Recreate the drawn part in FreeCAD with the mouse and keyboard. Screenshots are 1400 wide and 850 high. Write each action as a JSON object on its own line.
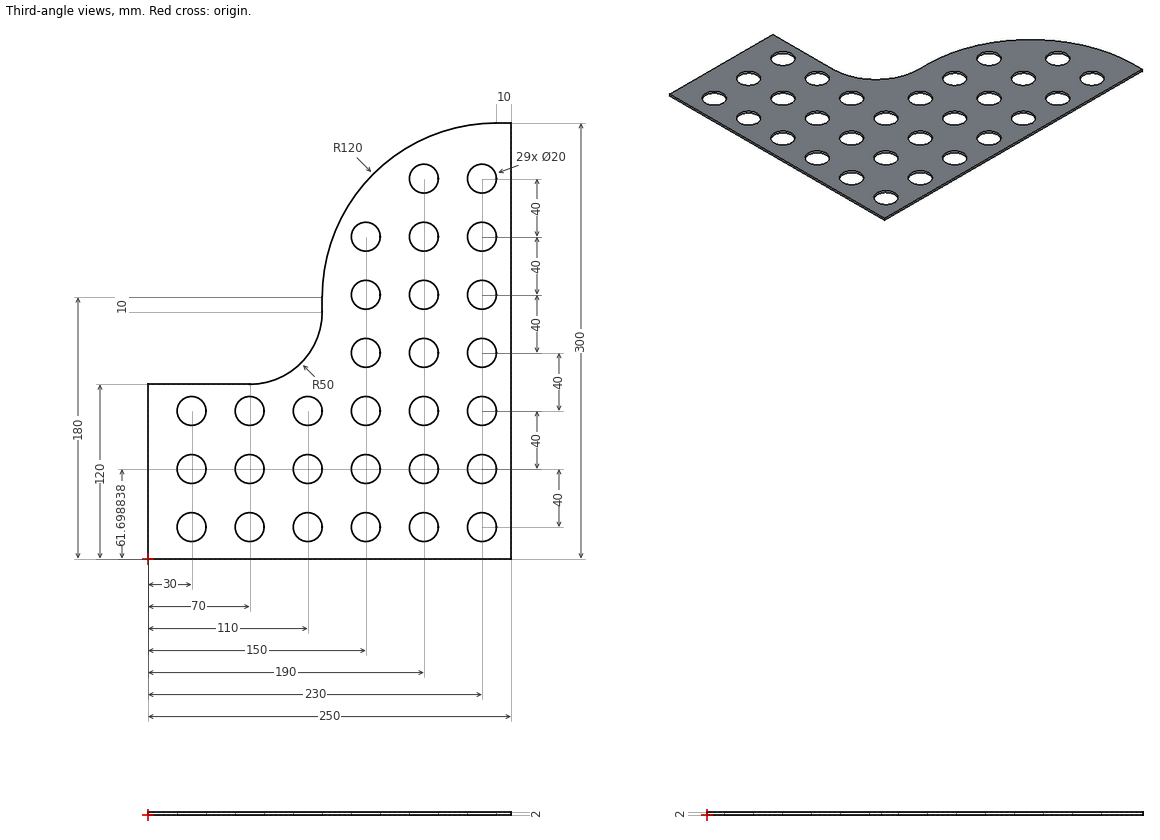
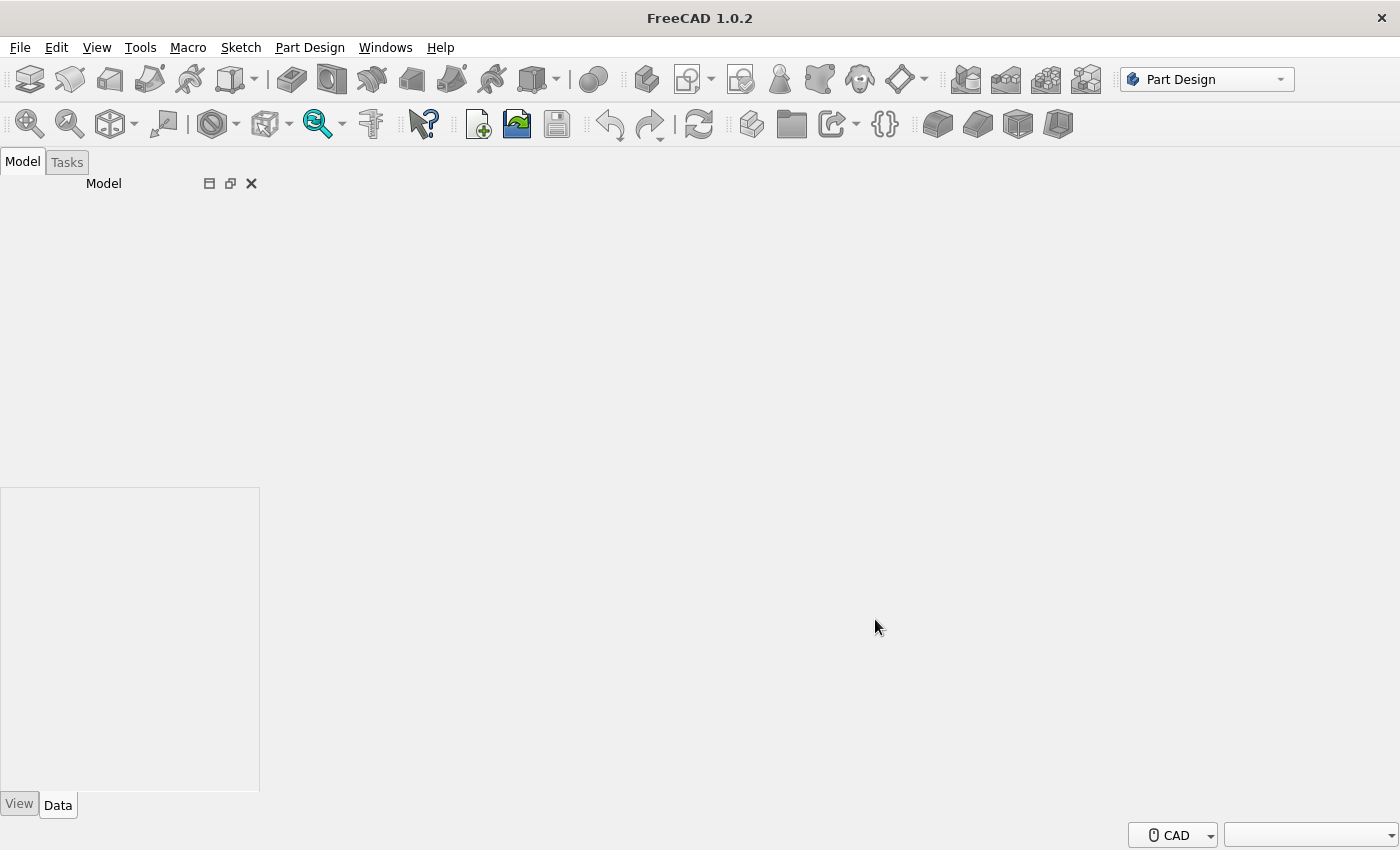
{"action": "left_click", "coordinate": [478, 124]}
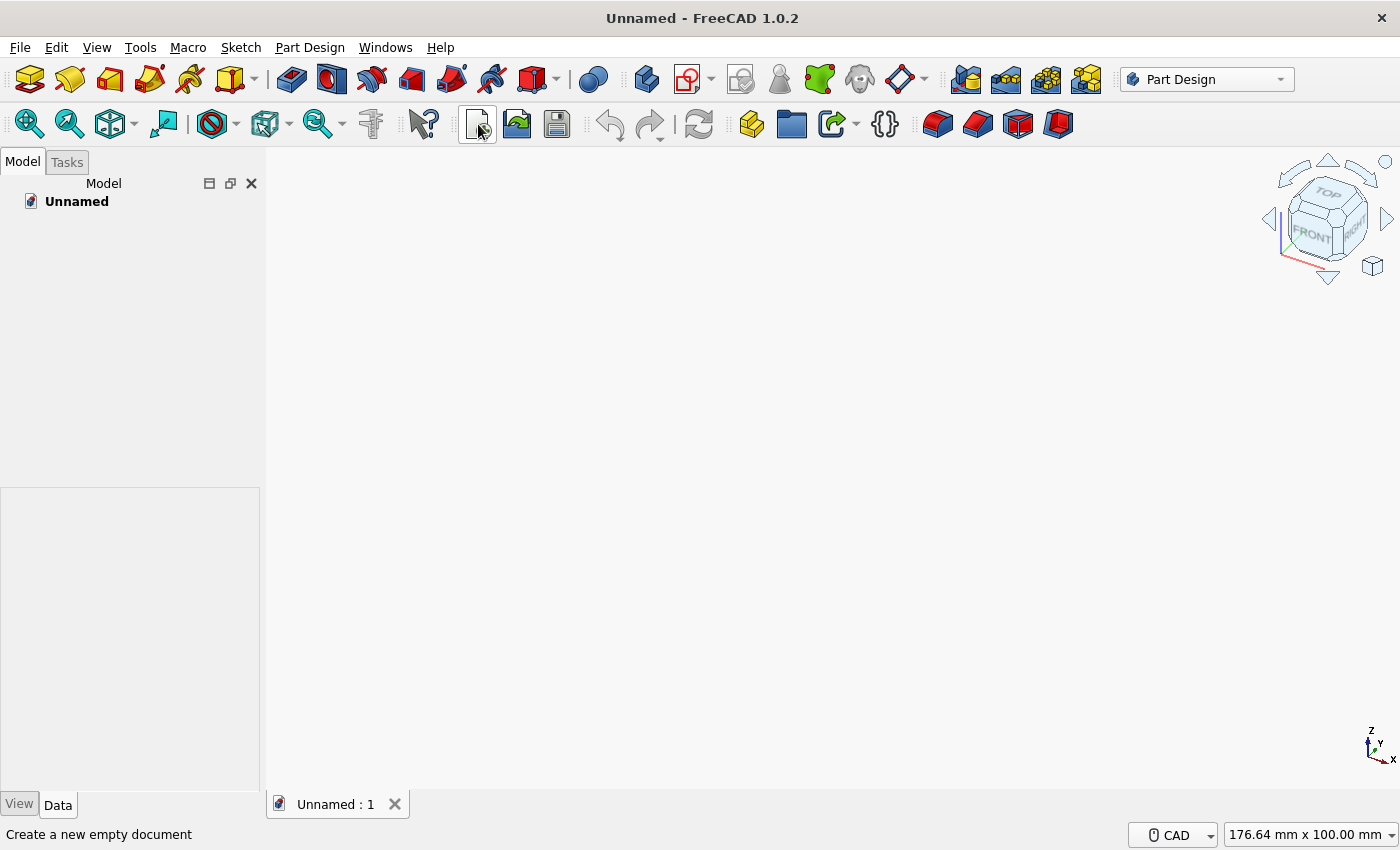
{"action": "left_click", "coordinate": [688, 80]}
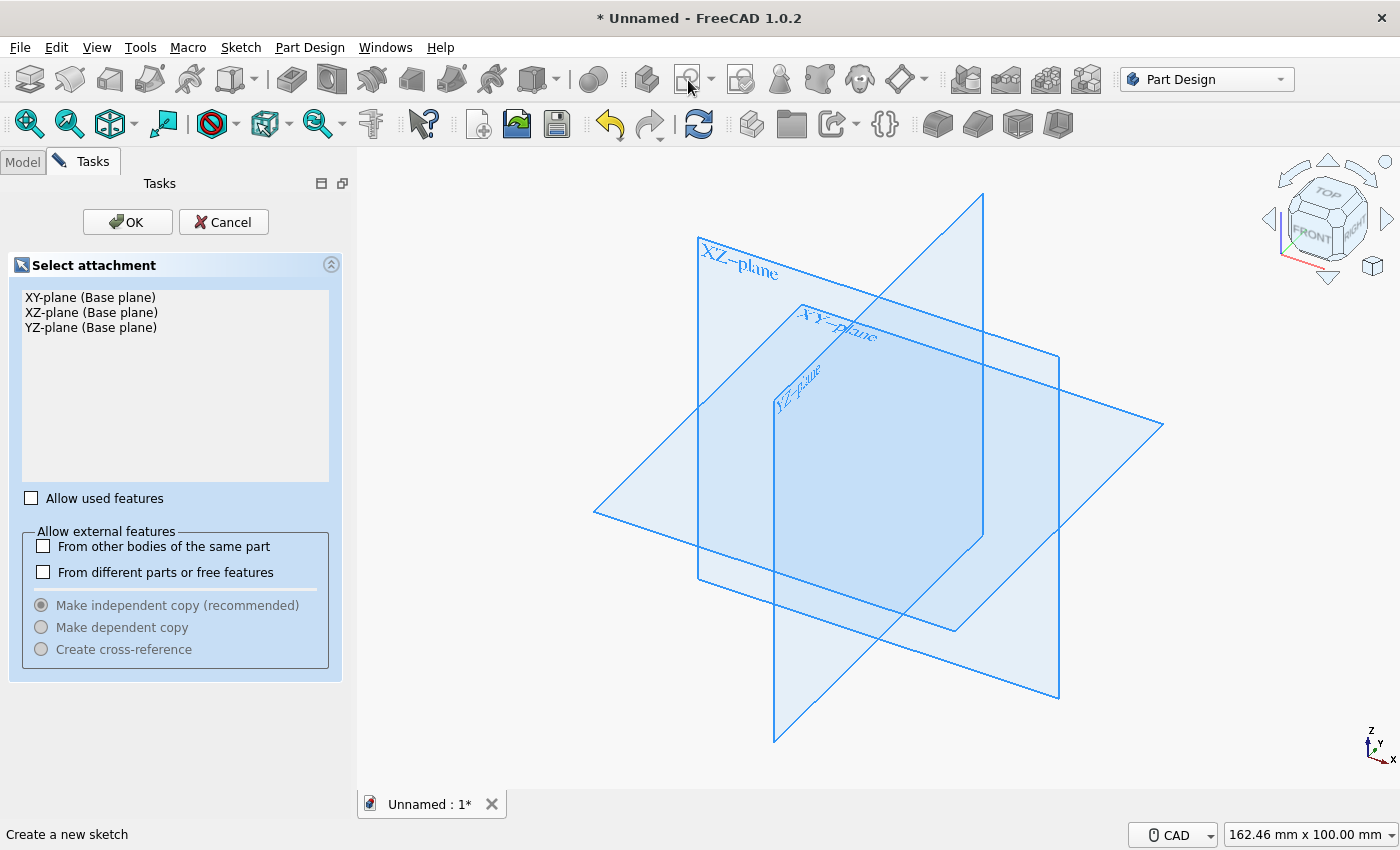
{"action": "left_click", "coordinate": [82, 298]}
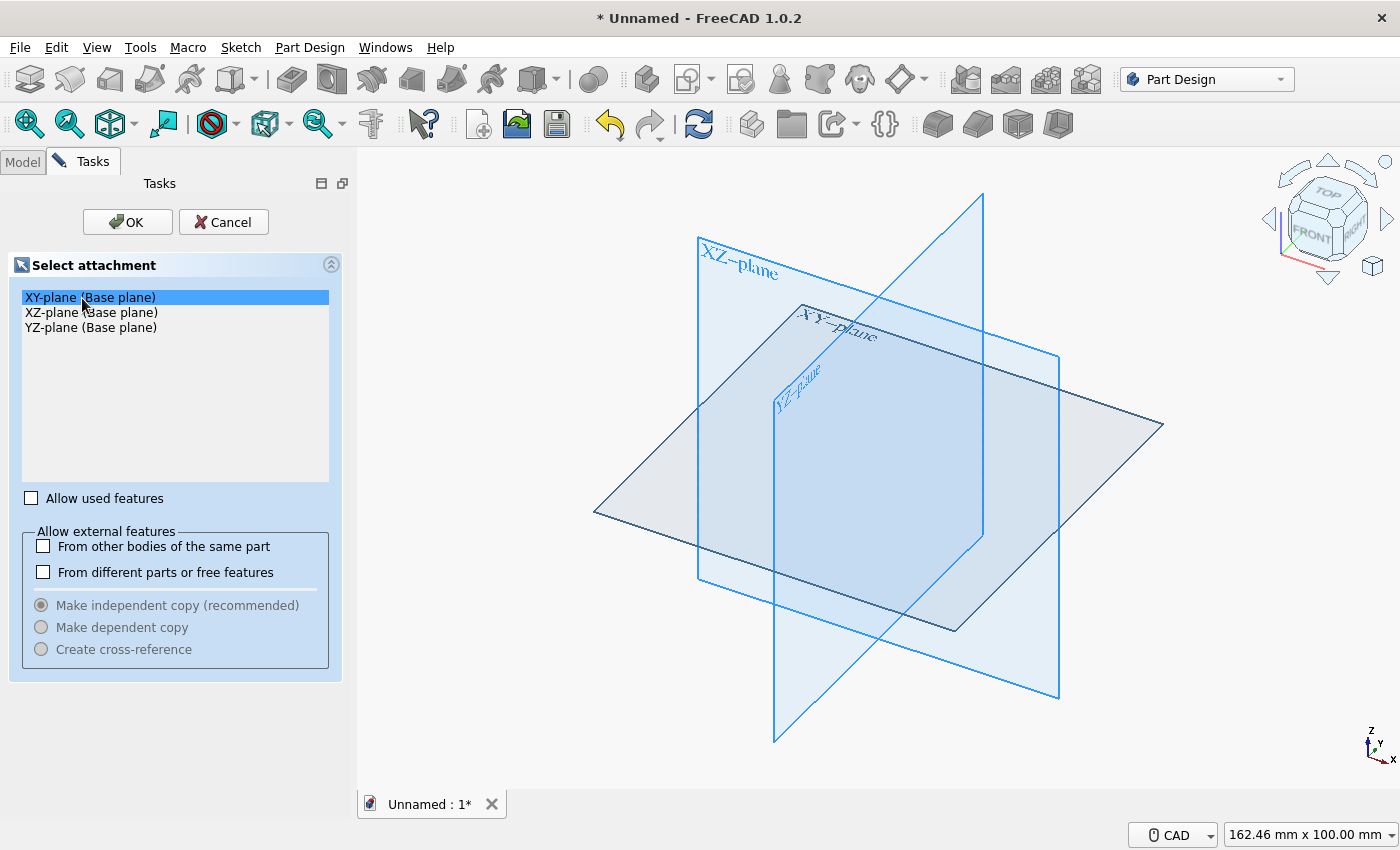
{"action": "left_click", "coordinate": [128, 222]}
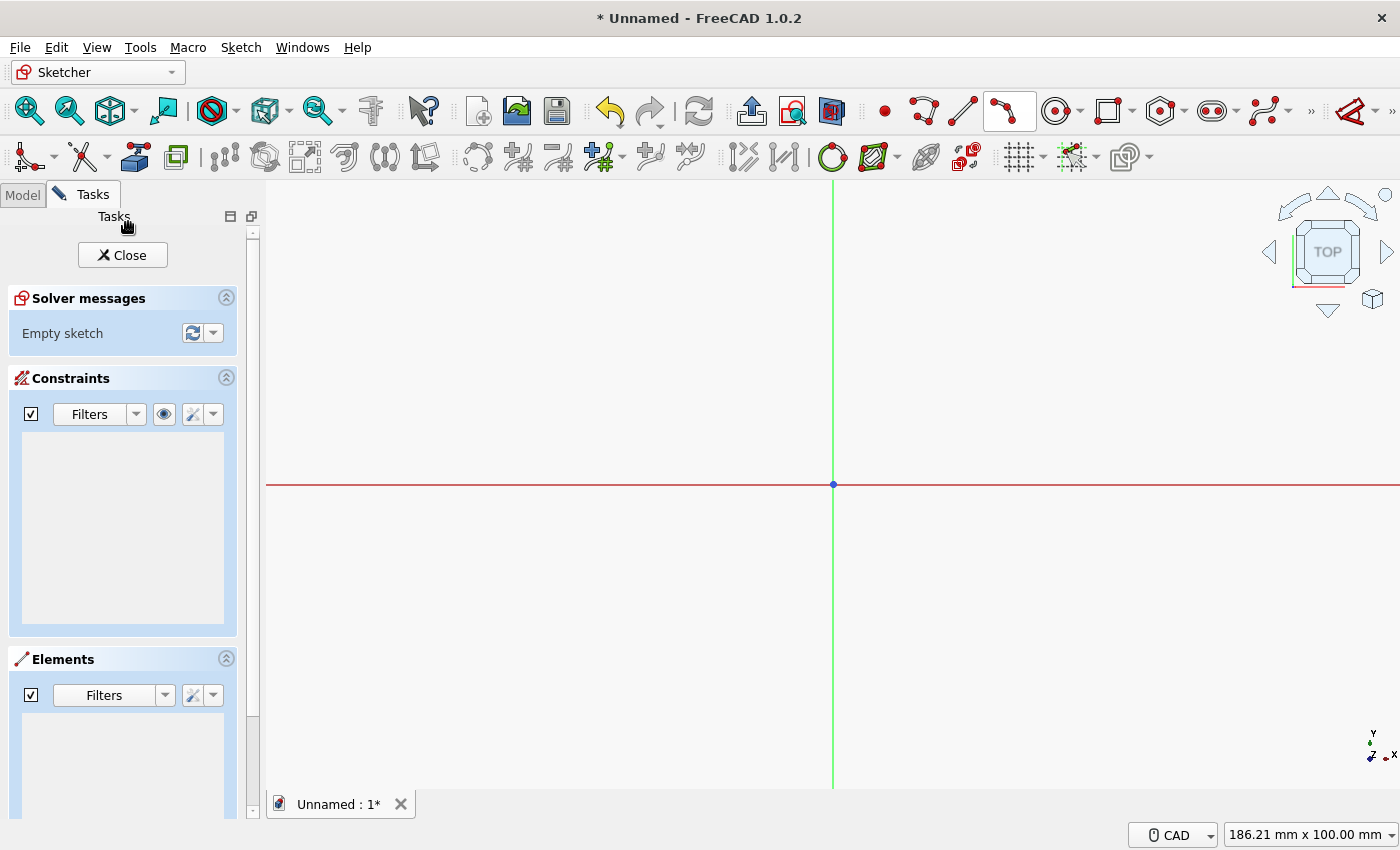
{"action": "scroll", "coordinate": [555, 716], "scroll_direction": "down", "scroll_amount": 8}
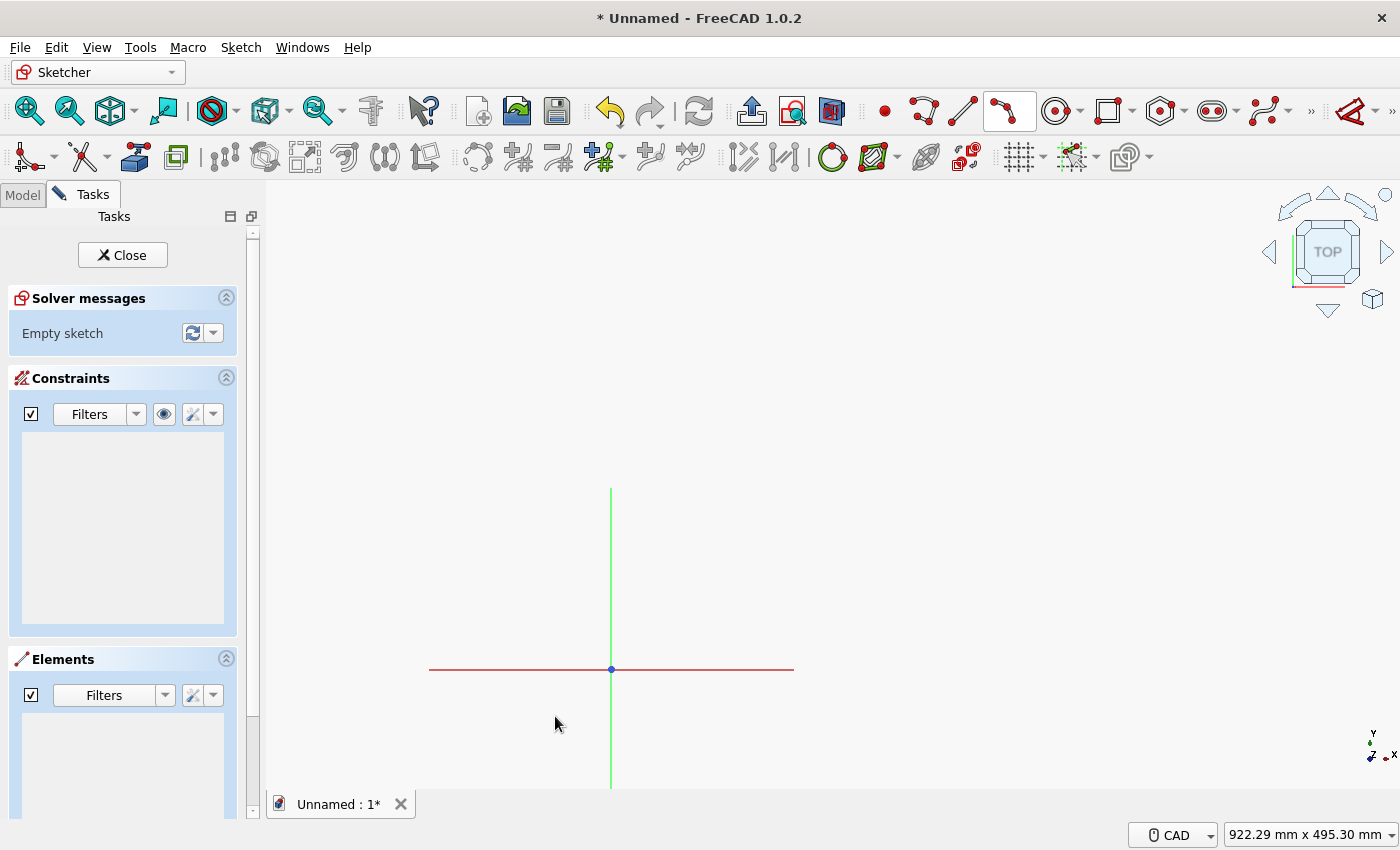
{"action": "left_click", "coordinate": [964, 112]}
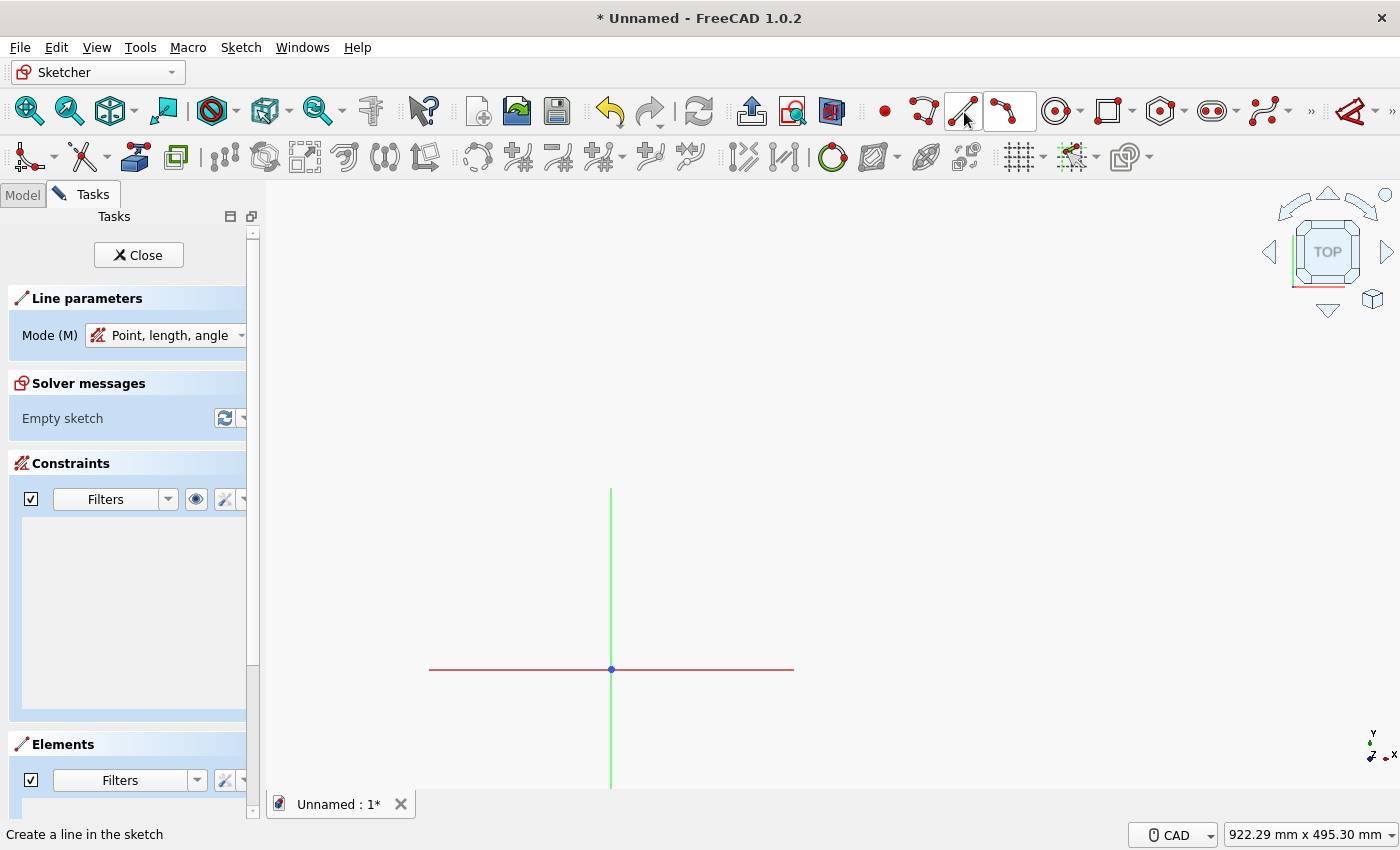
{"action": "left_click", "coordinate": [759, 449]}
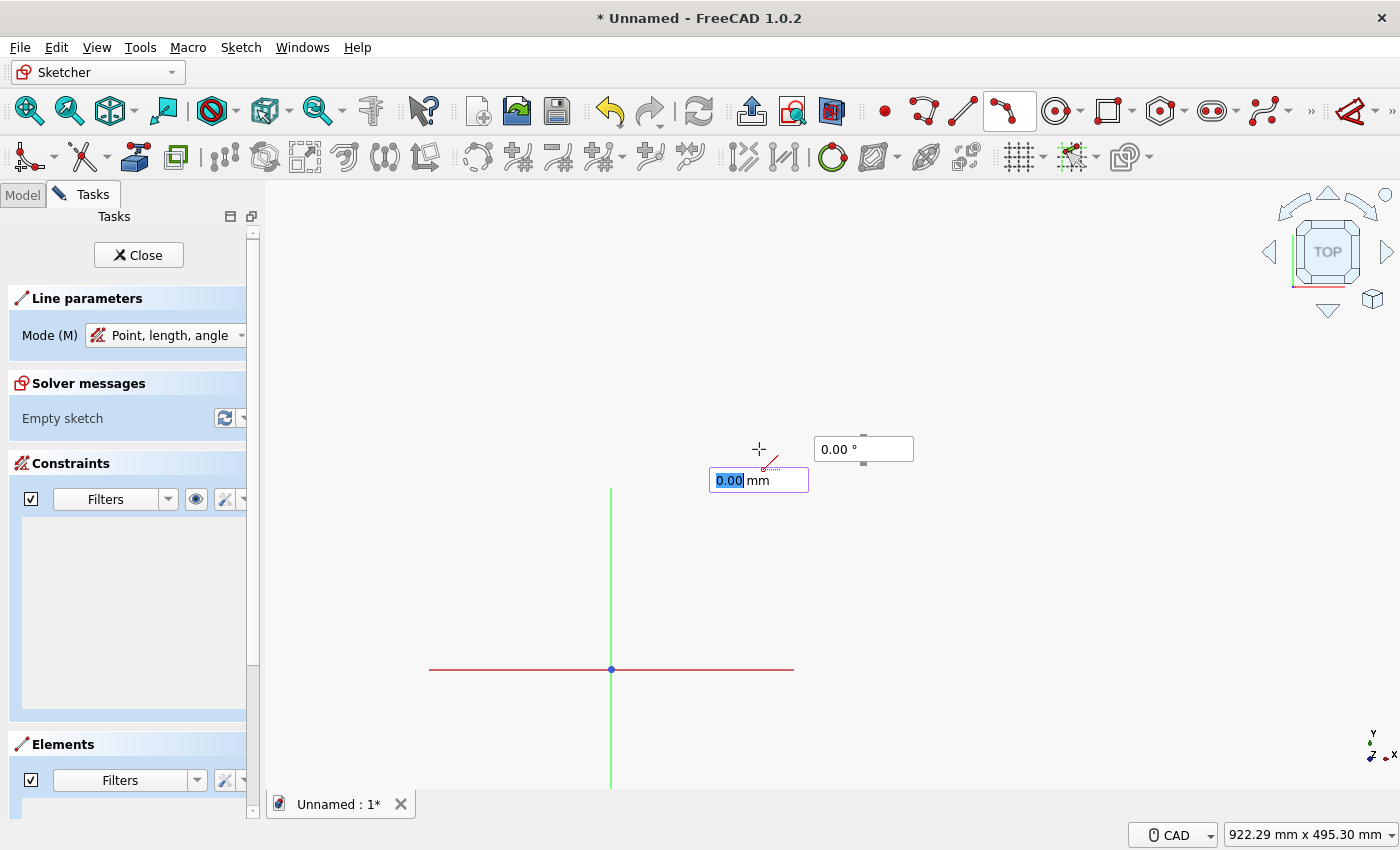
{"action": "scroll", "coordinate": [759, 461], "scroll_direction": "up", "scroll_amount": 2}